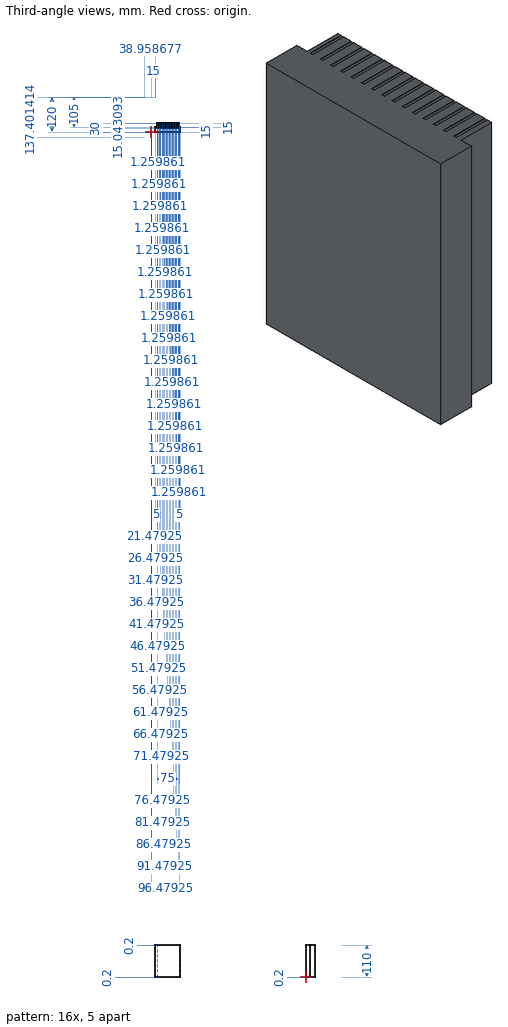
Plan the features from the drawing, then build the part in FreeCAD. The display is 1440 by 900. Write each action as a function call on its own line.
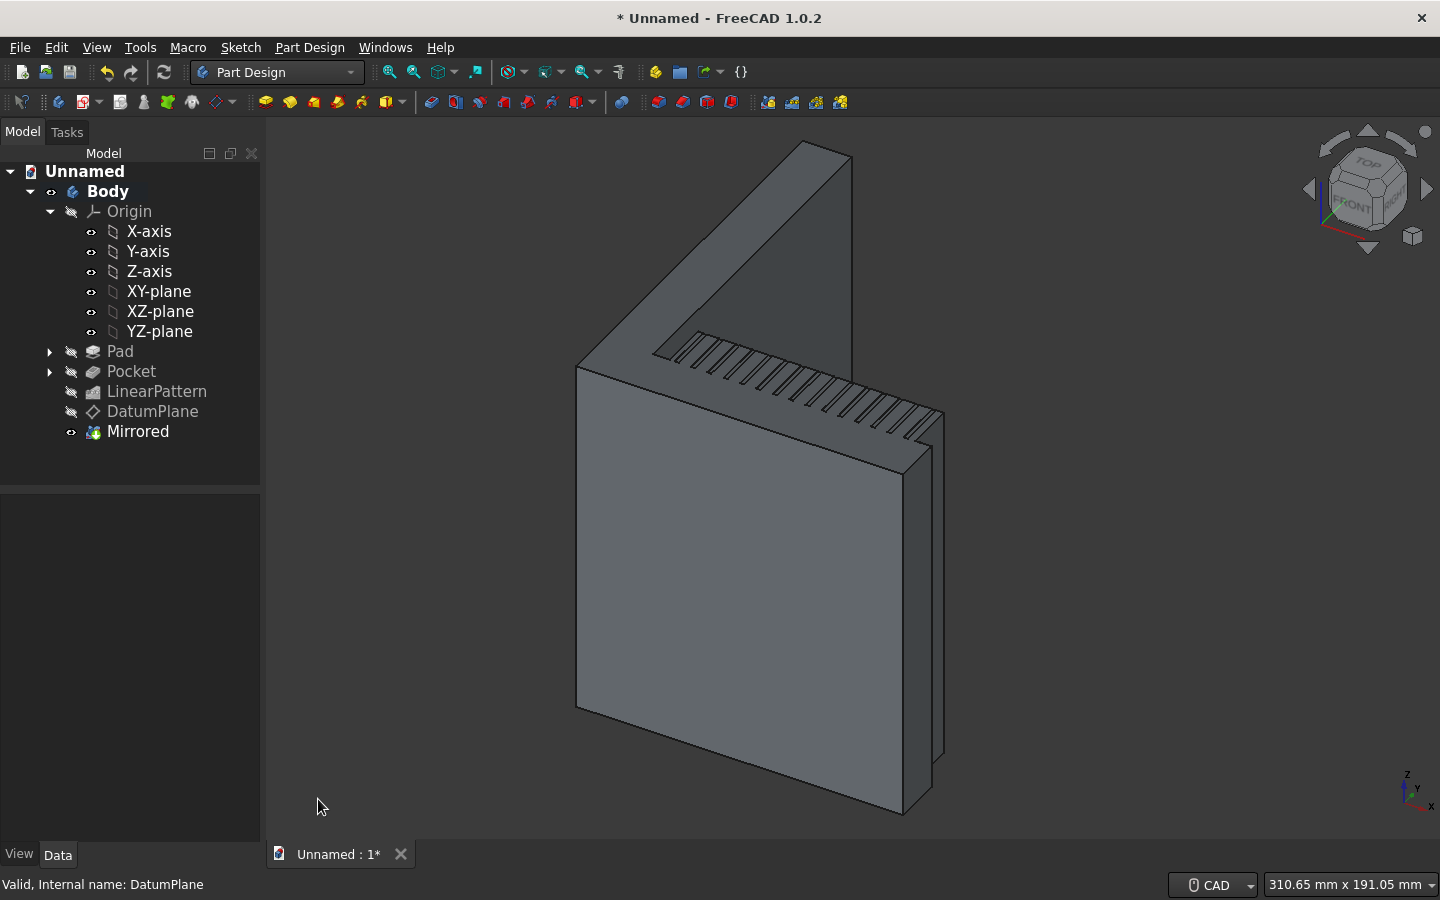
click(84, 102)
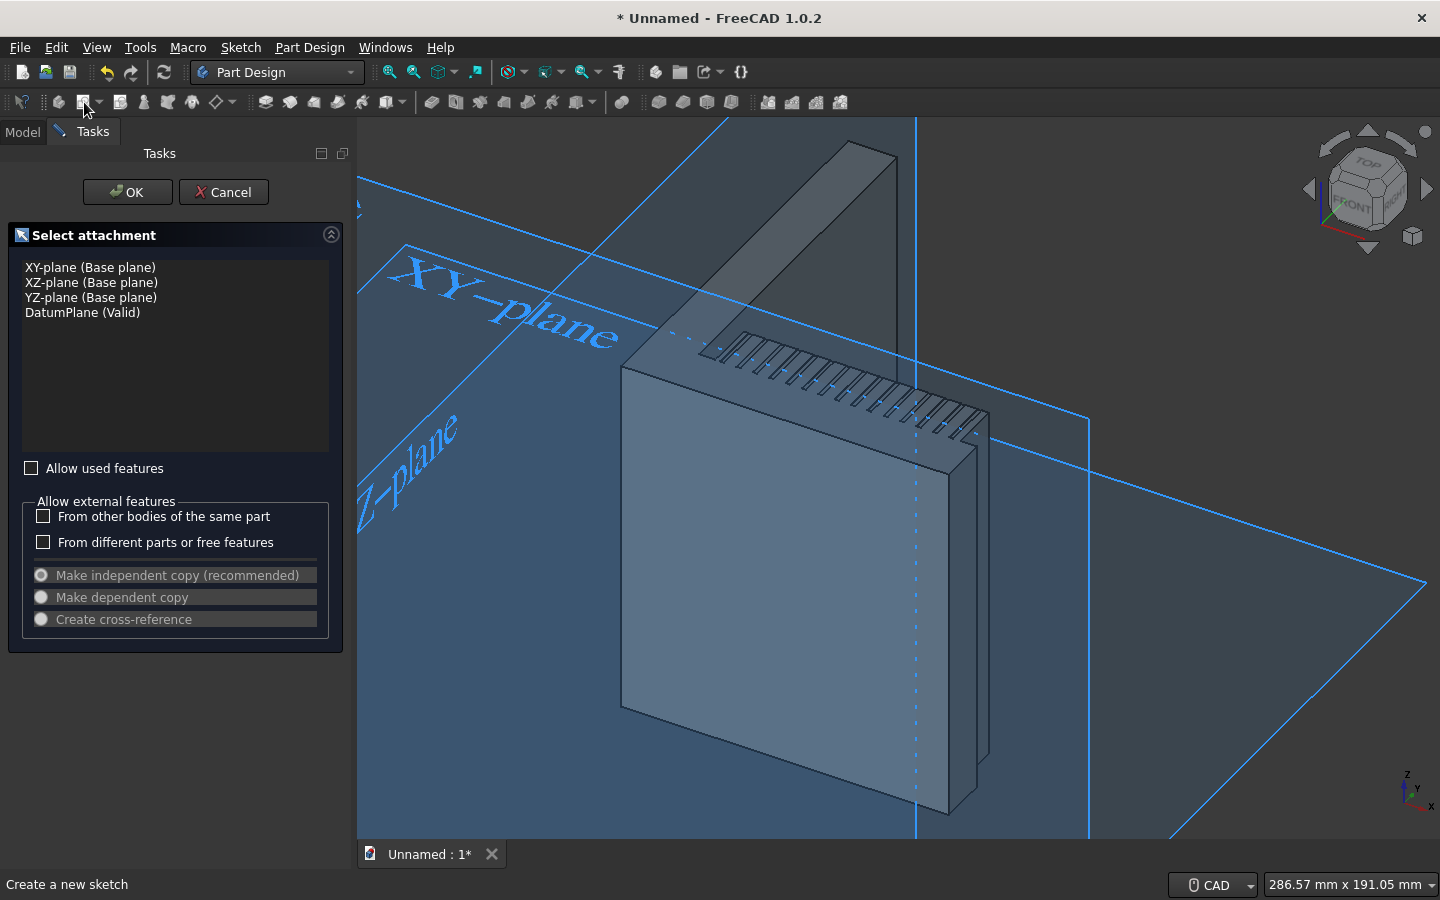
click(82, 268)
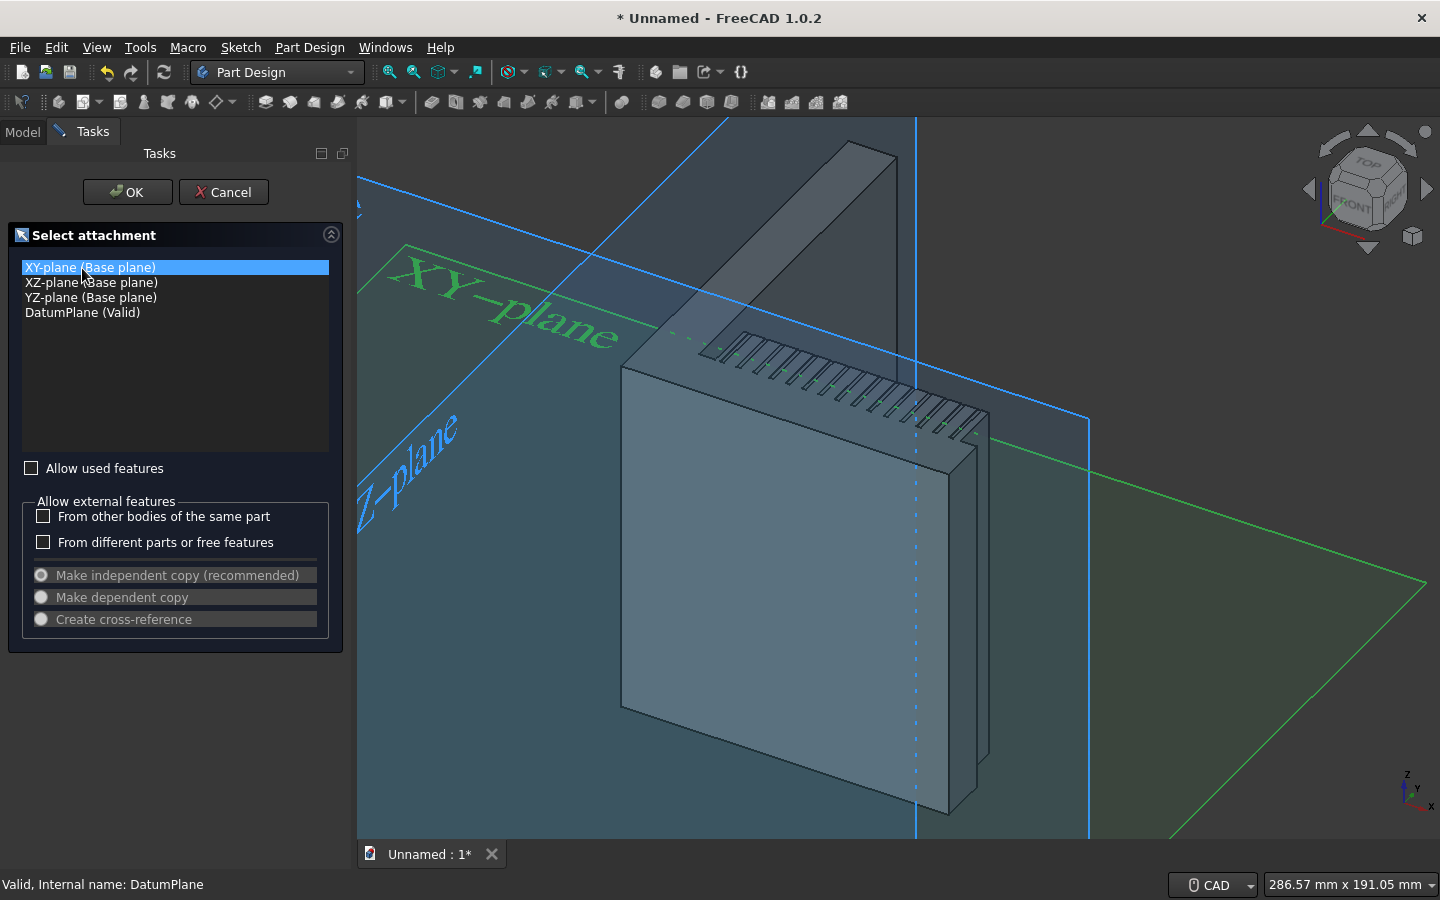
click(128, 192)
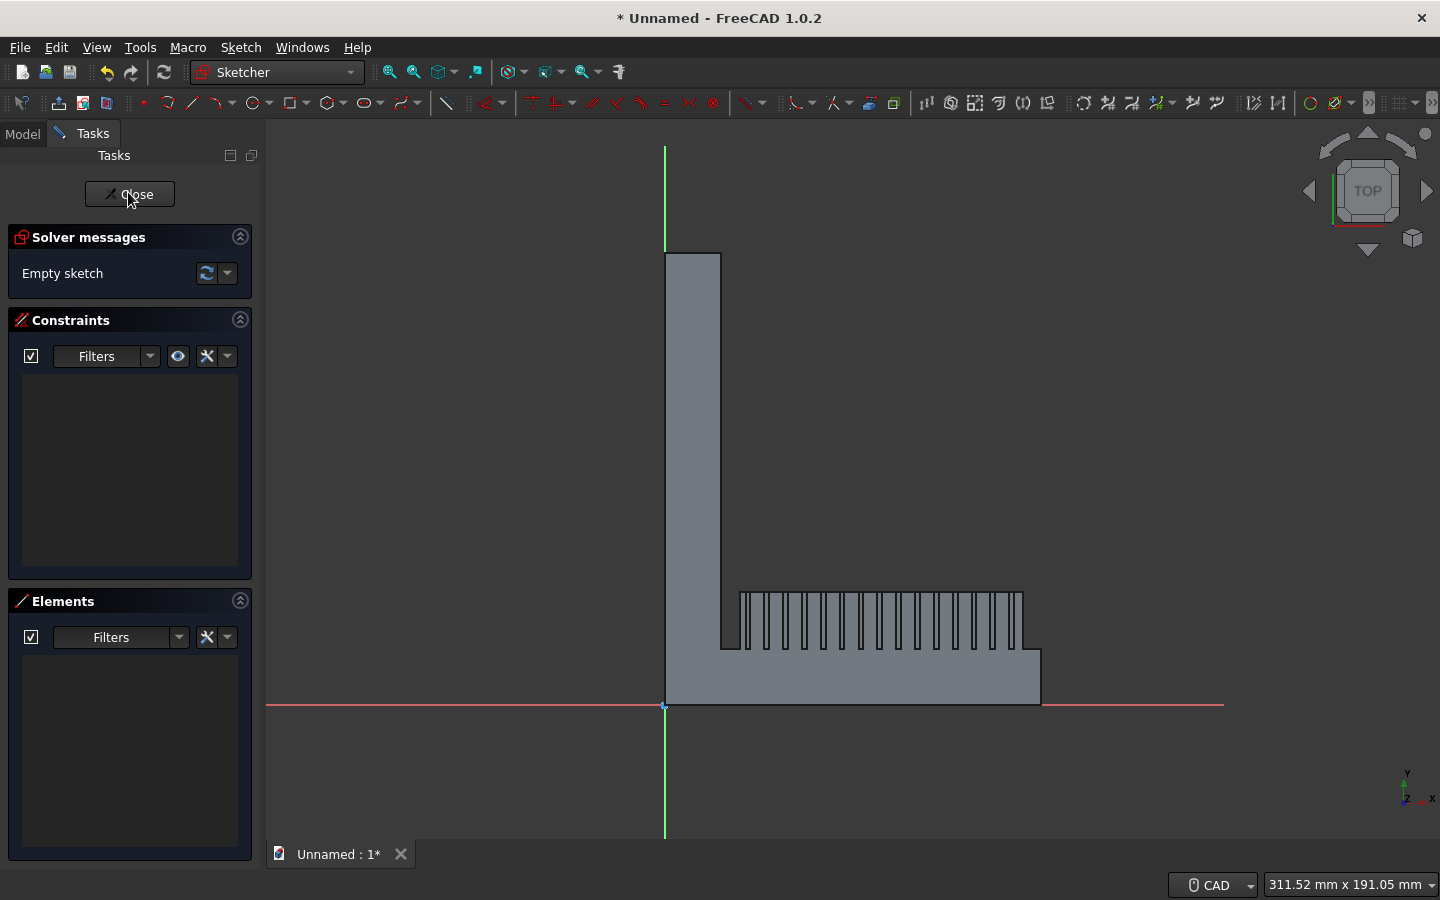
click(108, 104)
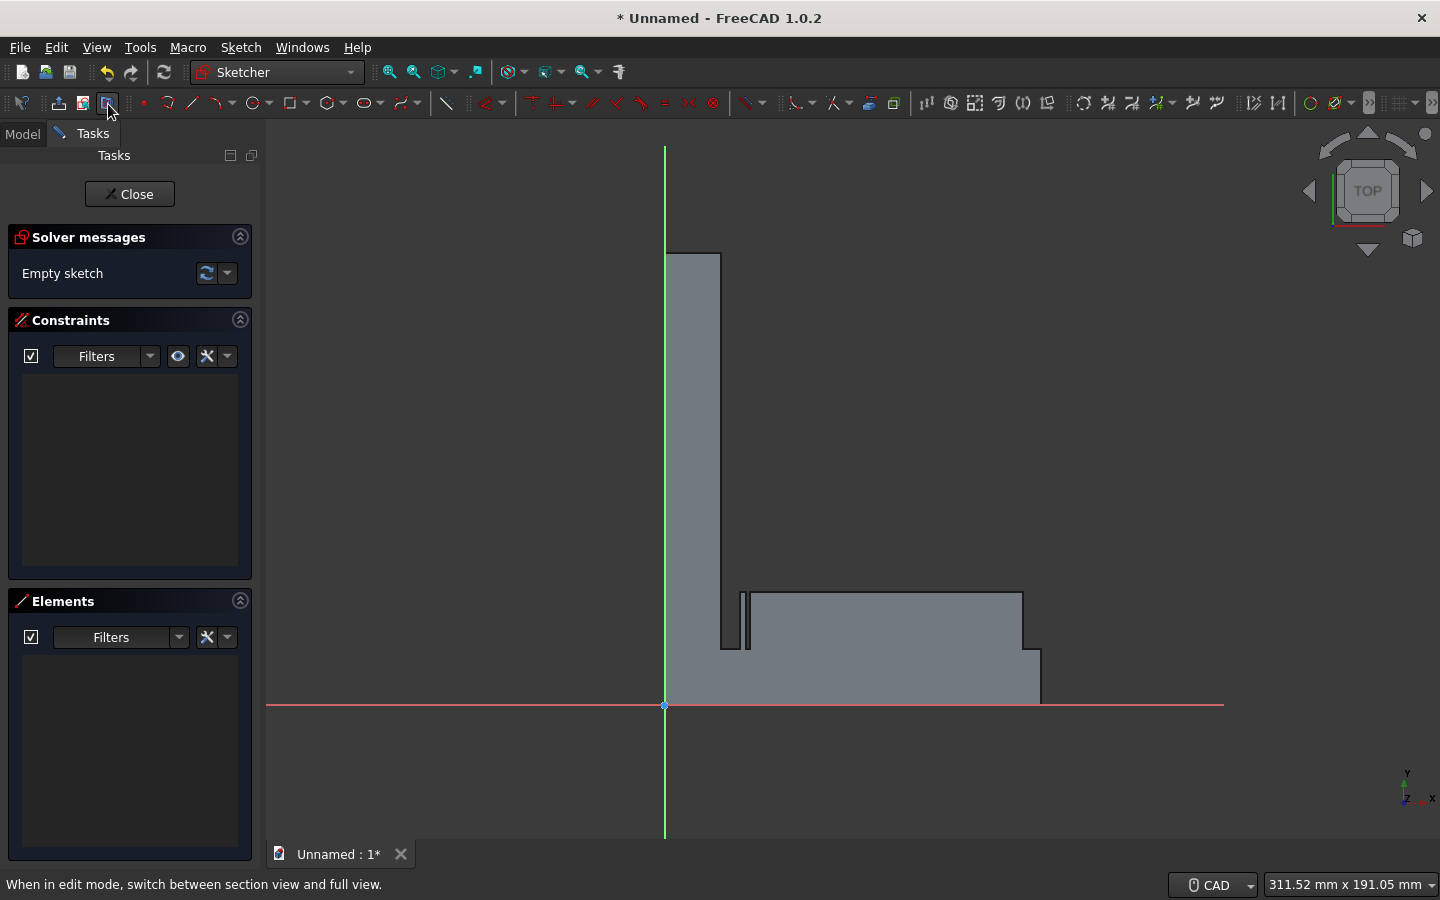
scroll(695, 704, up, 7)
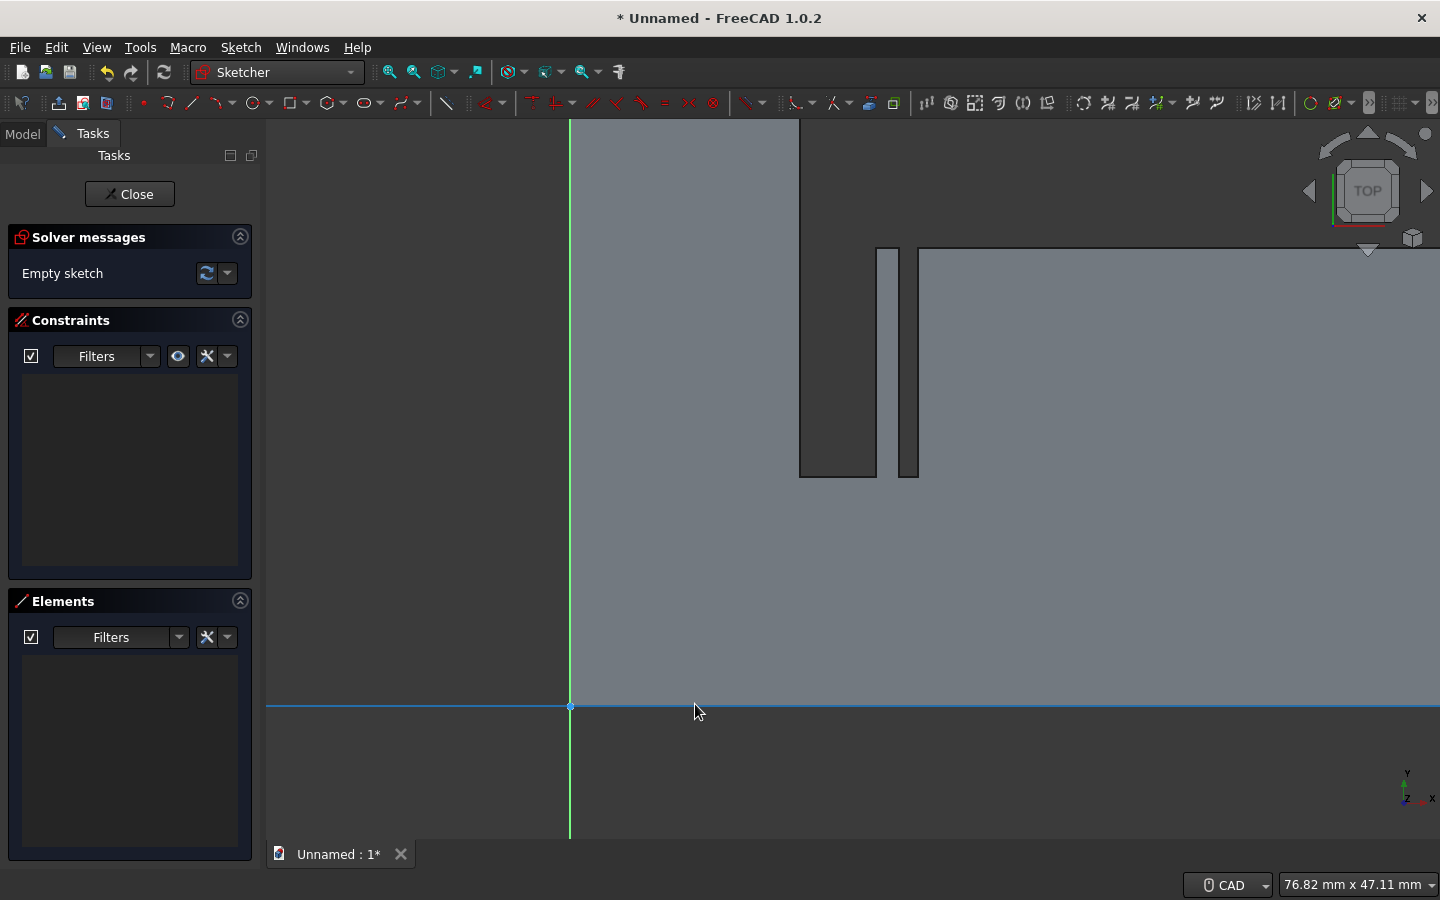
click(290, 104)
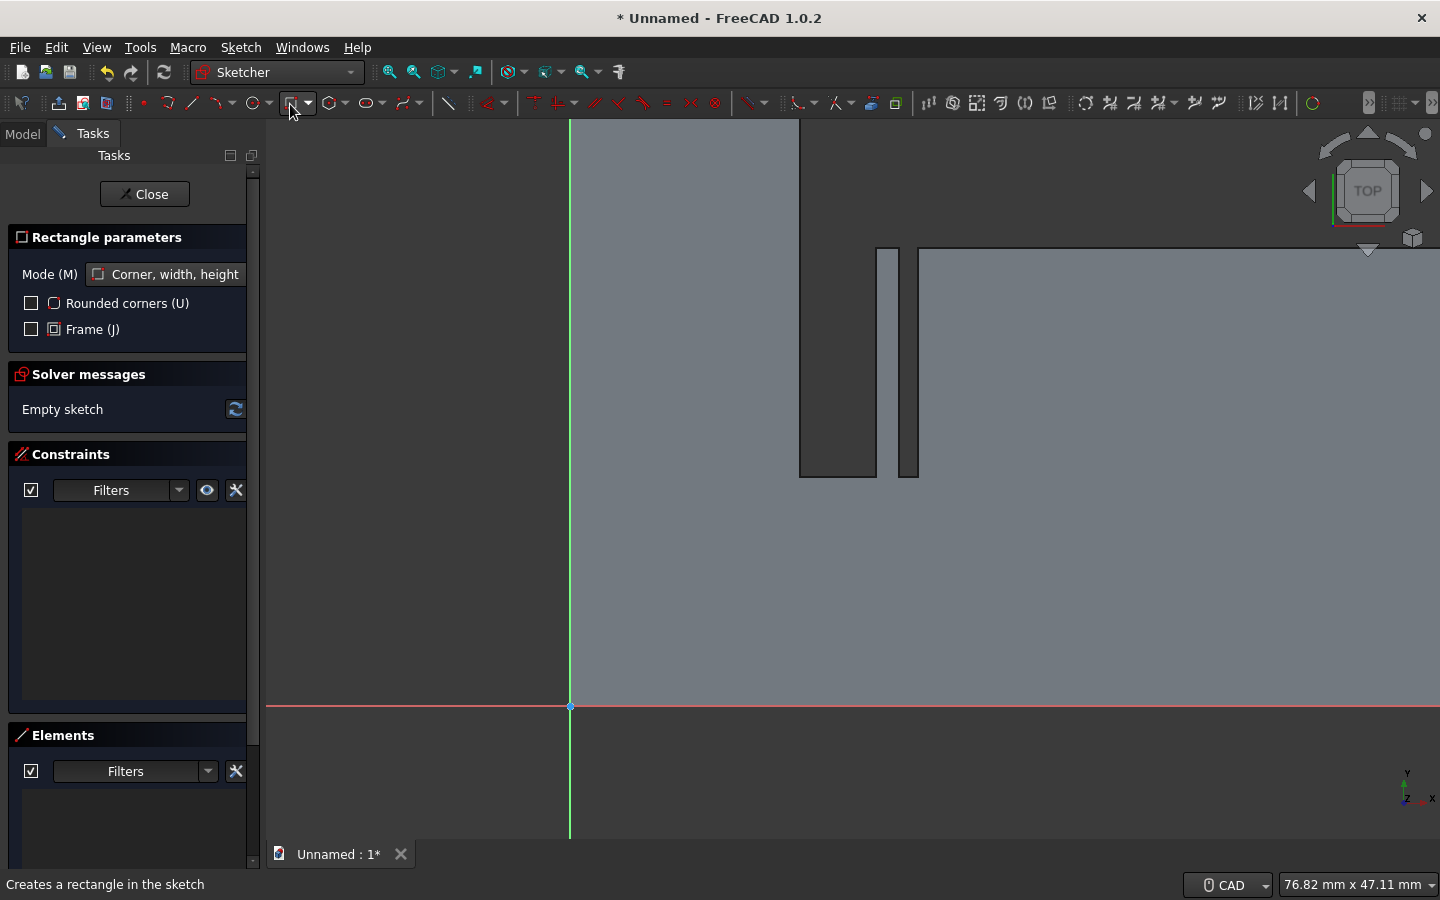
click(975, 248)
click(994, 477)
key(Escape)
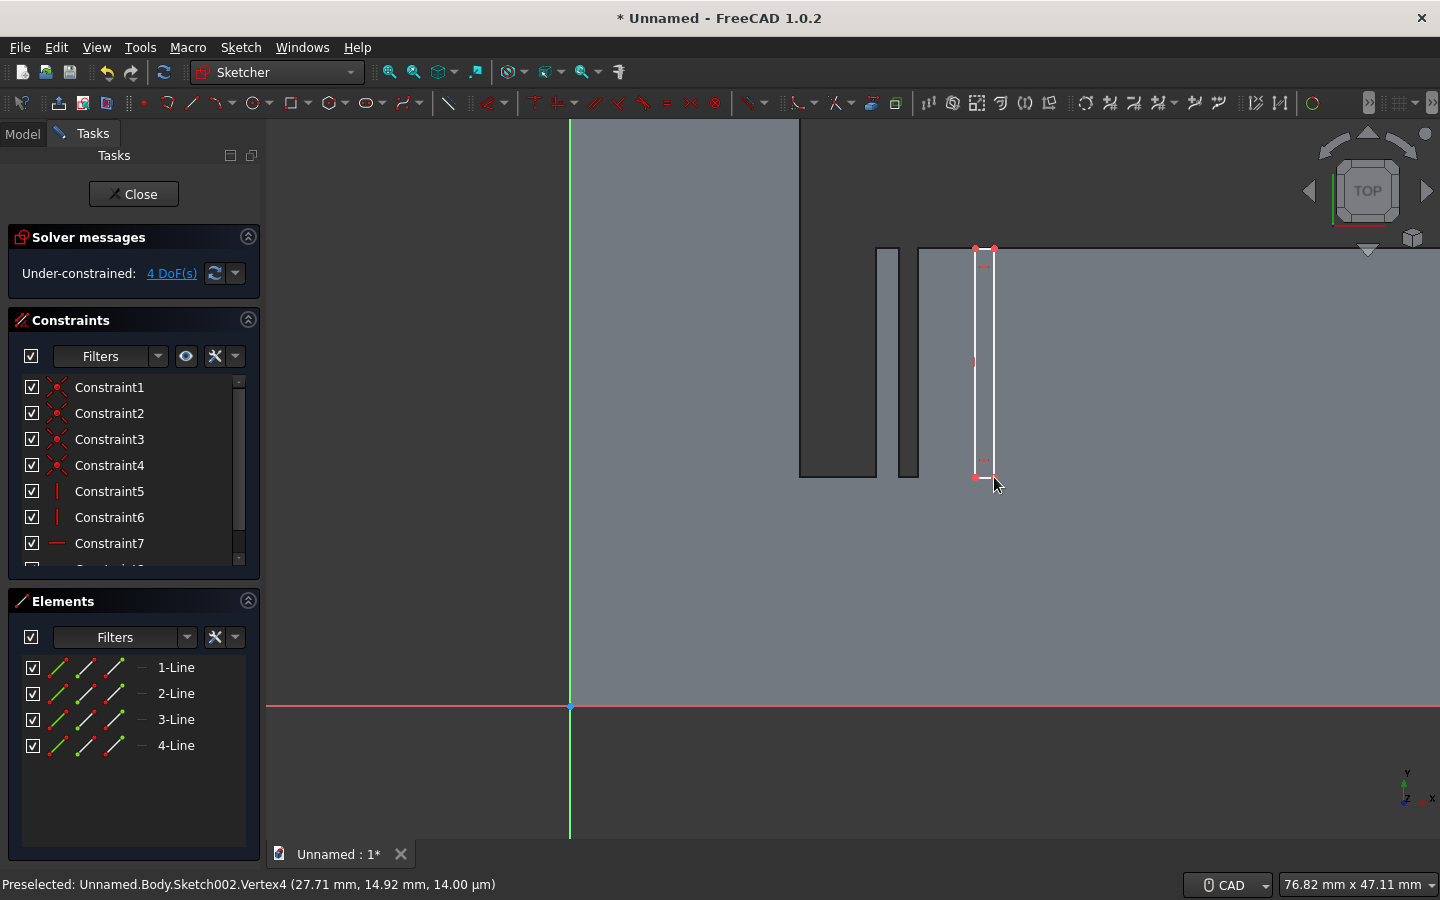
key(d)